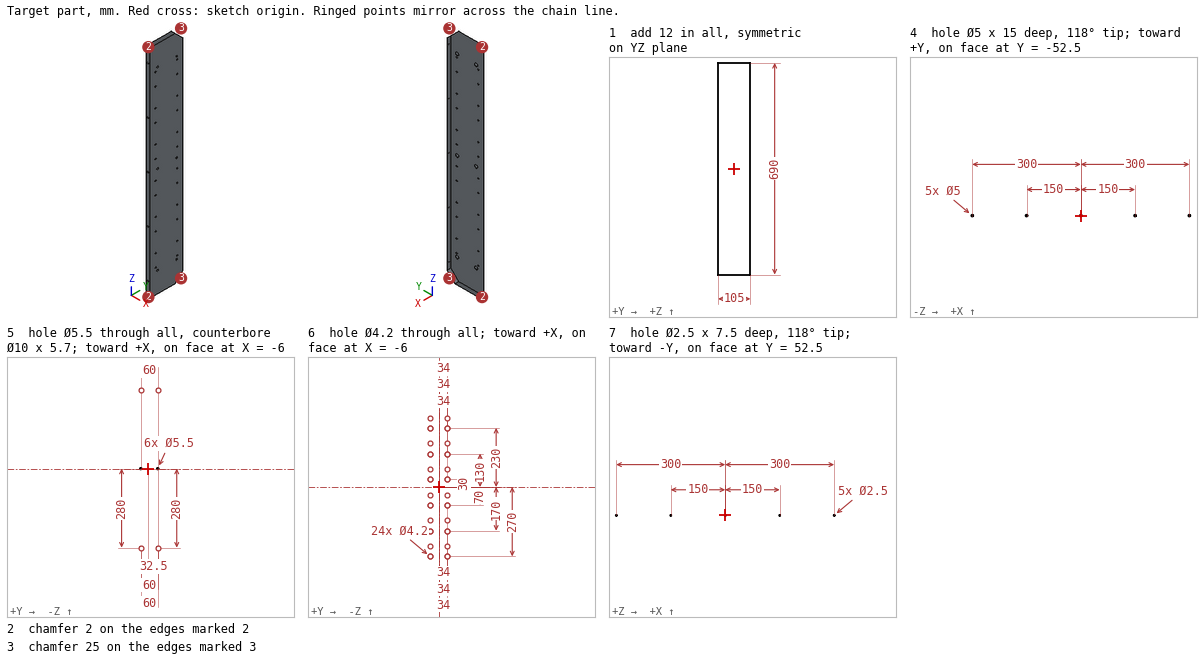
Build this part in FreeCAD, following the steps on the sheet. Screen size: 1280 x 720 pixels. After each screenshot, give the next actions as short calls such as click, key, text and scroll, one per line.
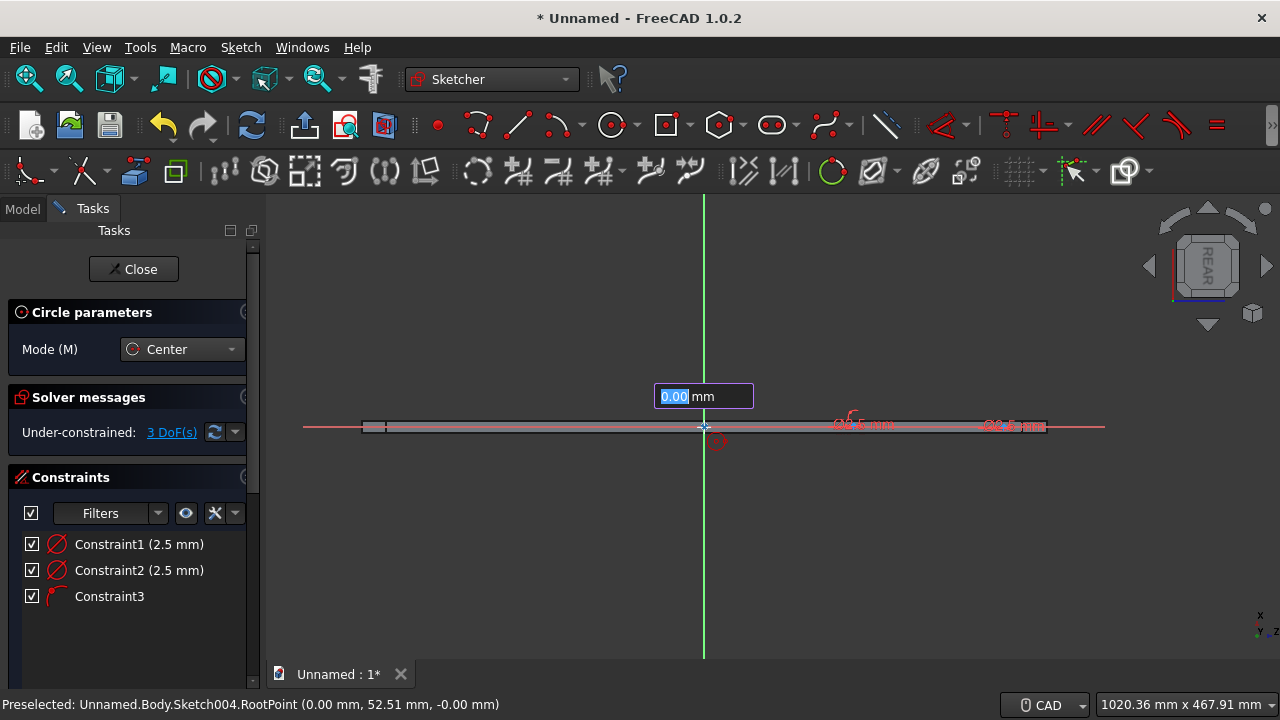
scroll(705, 426, up, 15)
move(703, 410)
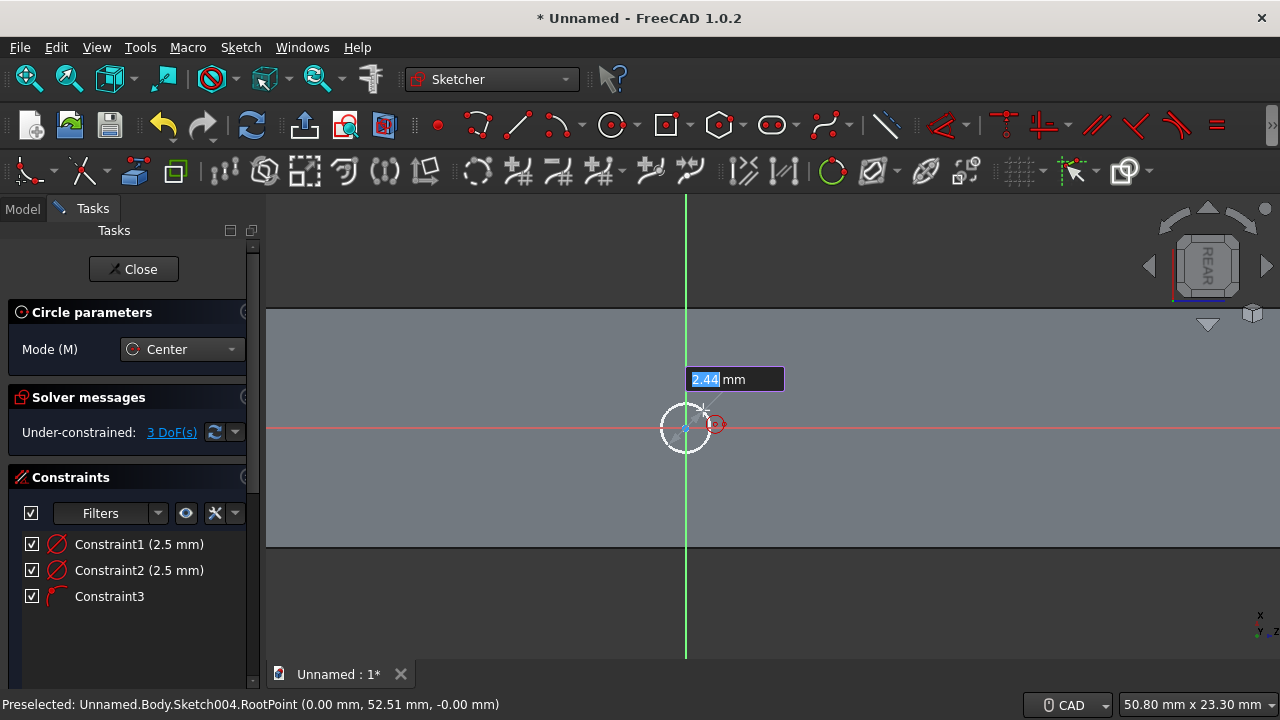
text(2.5)
key(Return)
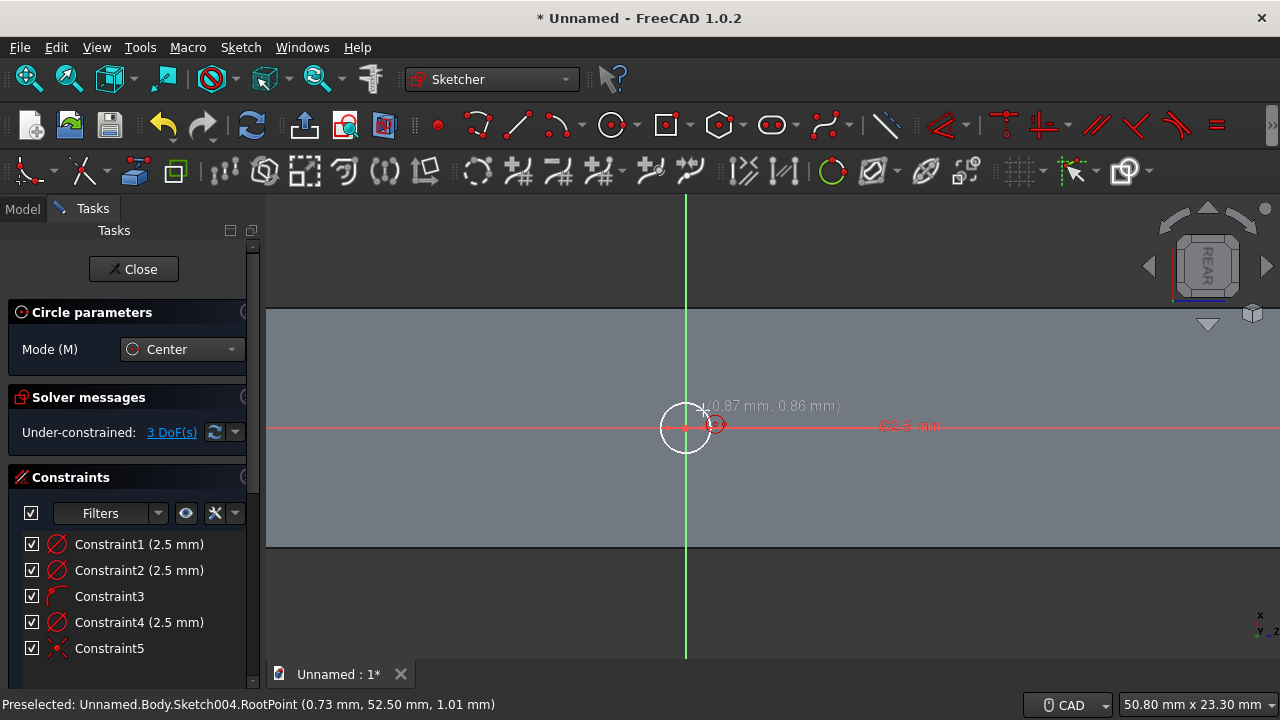
scroll(705, 426, down, 15)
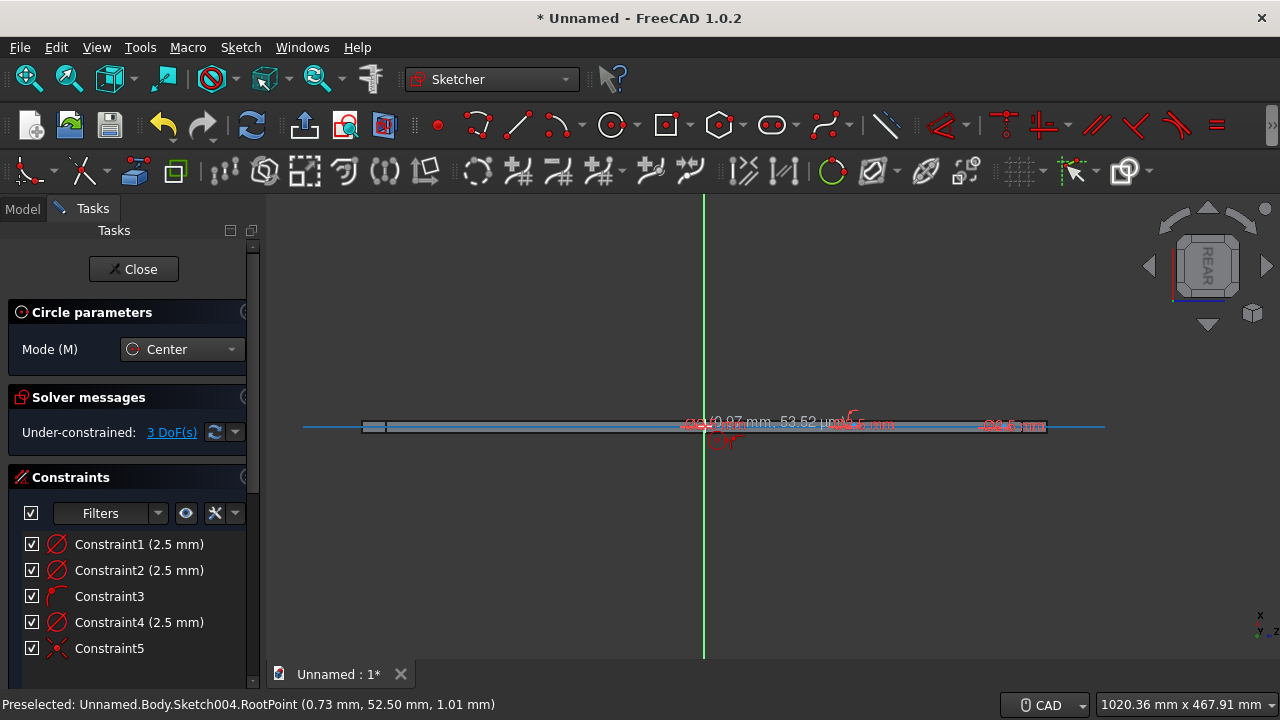
scroll(555, 427, up, 15)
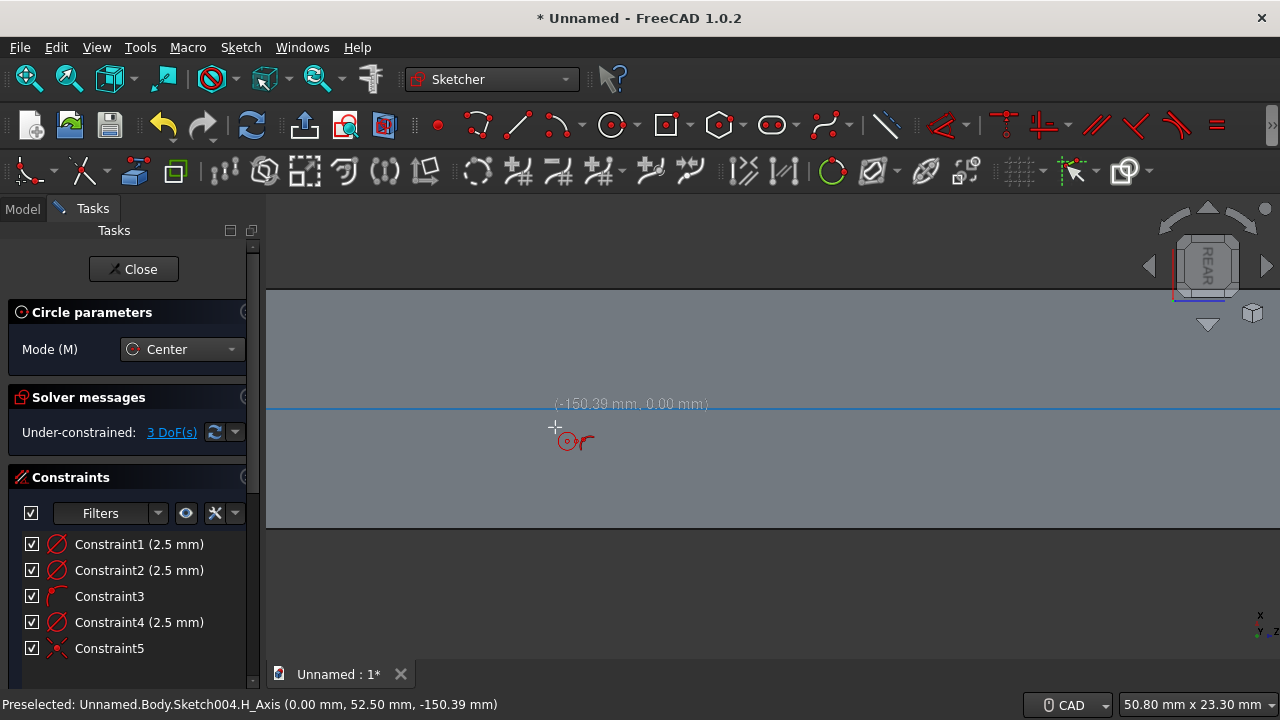
scroll(555, 427, down, 15)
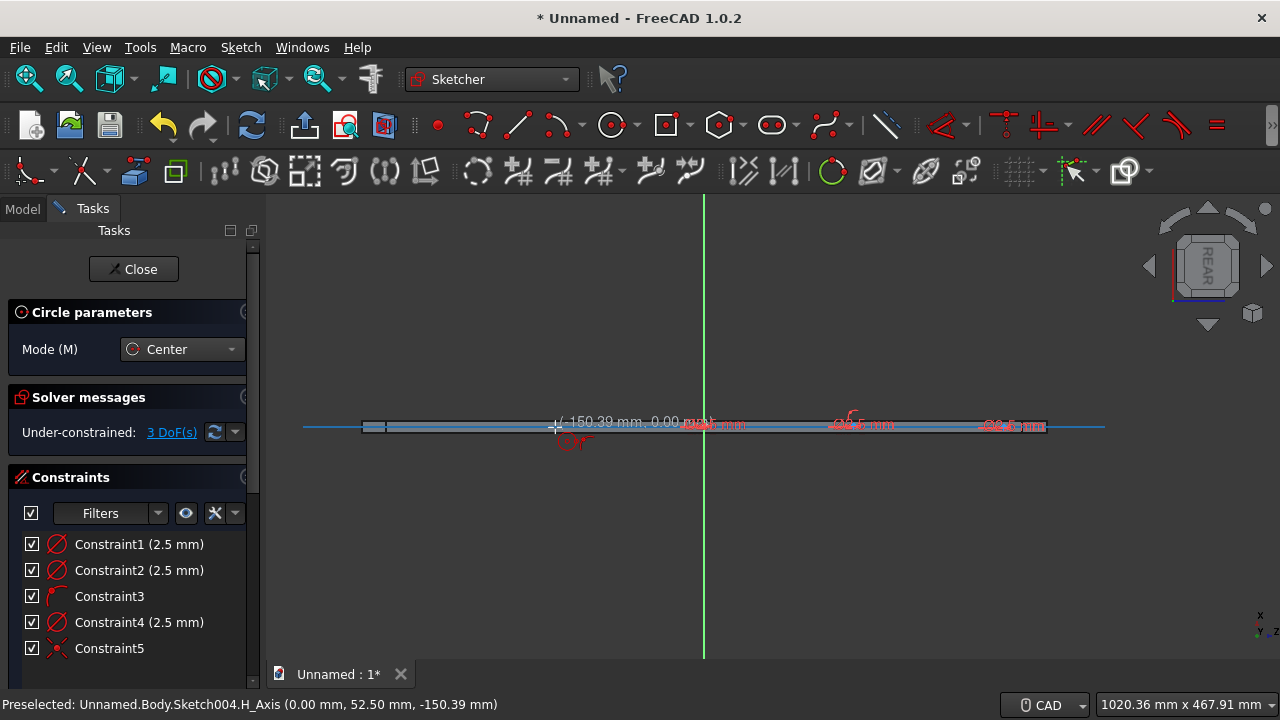
click(555, 427)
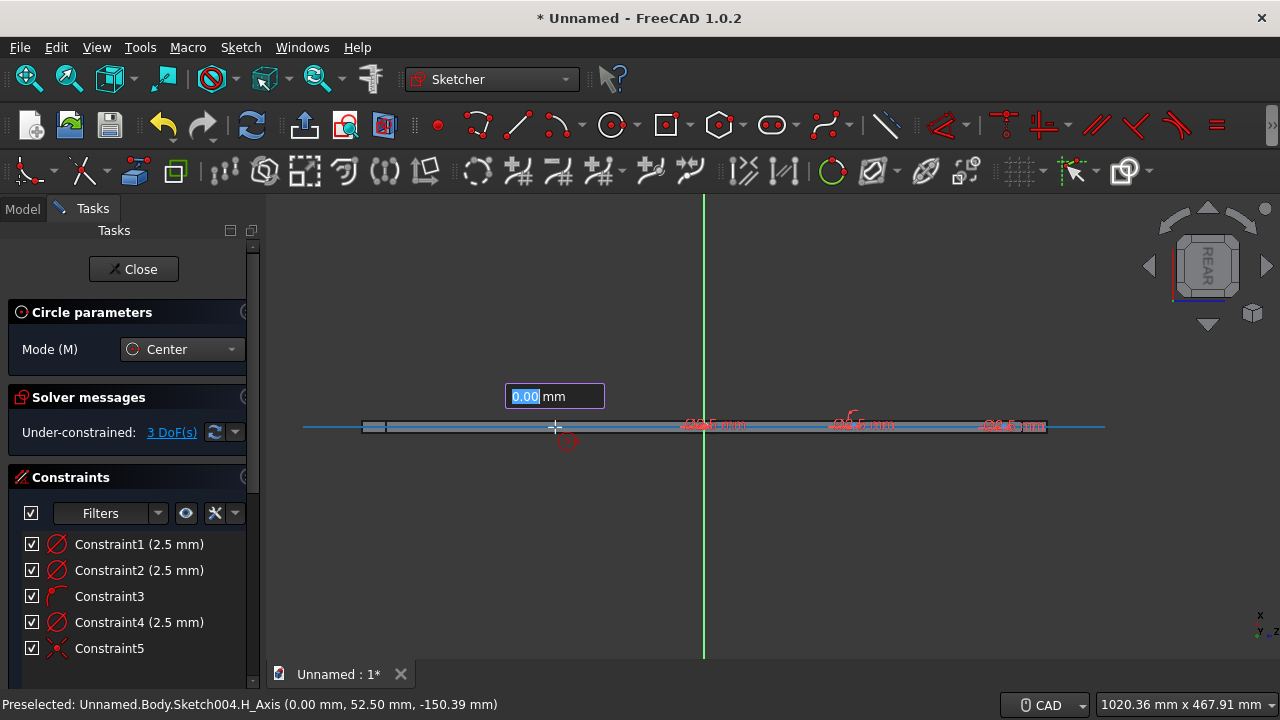
scroll(555, 428, up, 14)
move(550, 416)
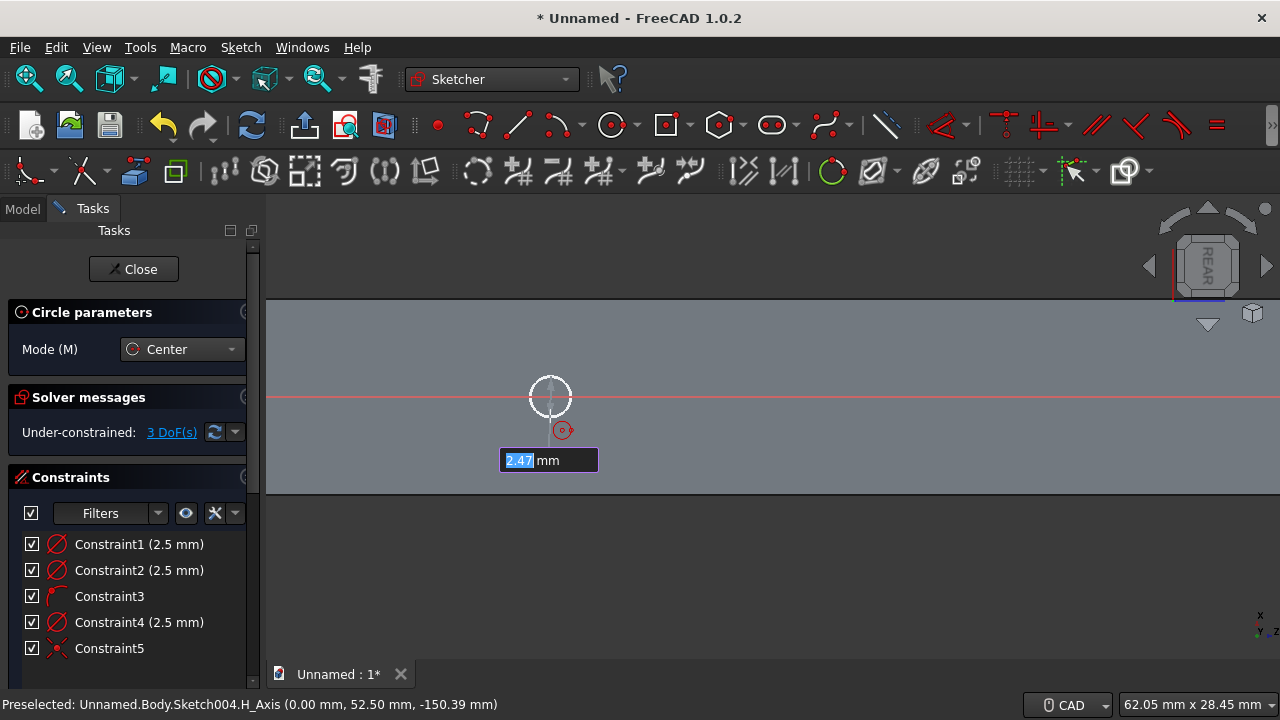
text(2.5)
key(Return)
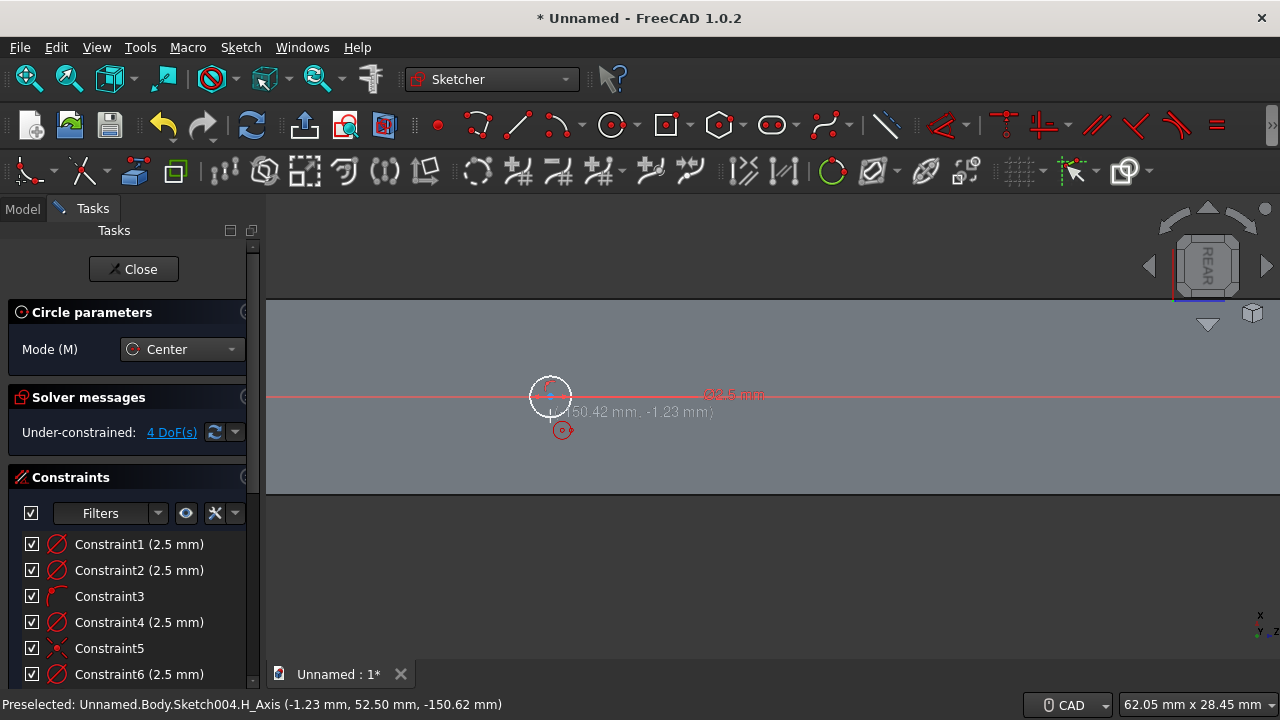
scroll(555, 428, down, 14)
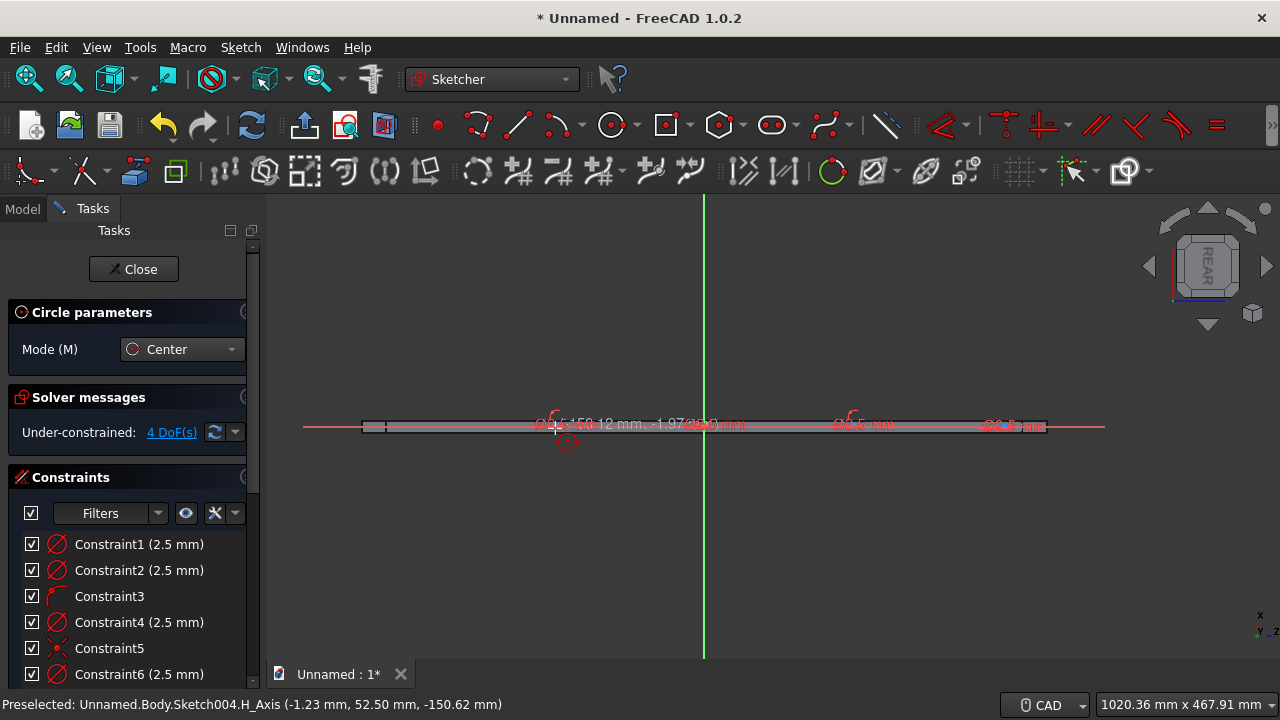
scroll(406, 427, up, 15)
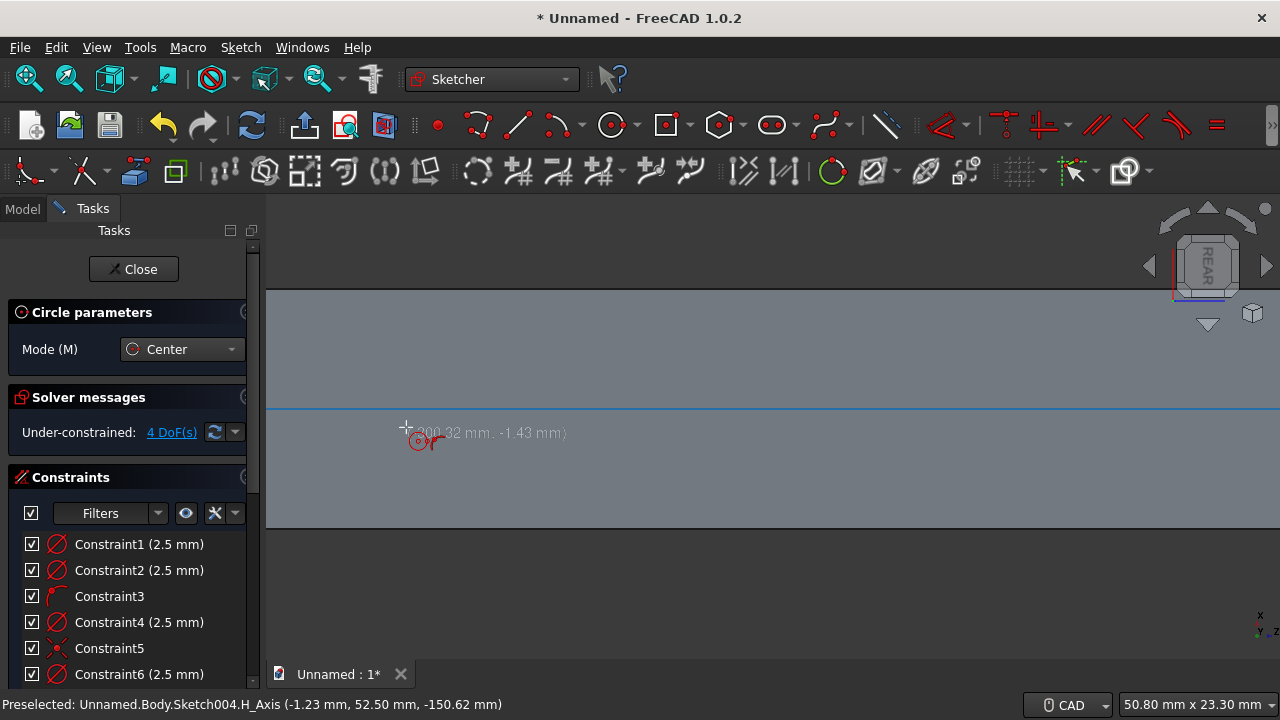
scroll(406, 427, down, 15)